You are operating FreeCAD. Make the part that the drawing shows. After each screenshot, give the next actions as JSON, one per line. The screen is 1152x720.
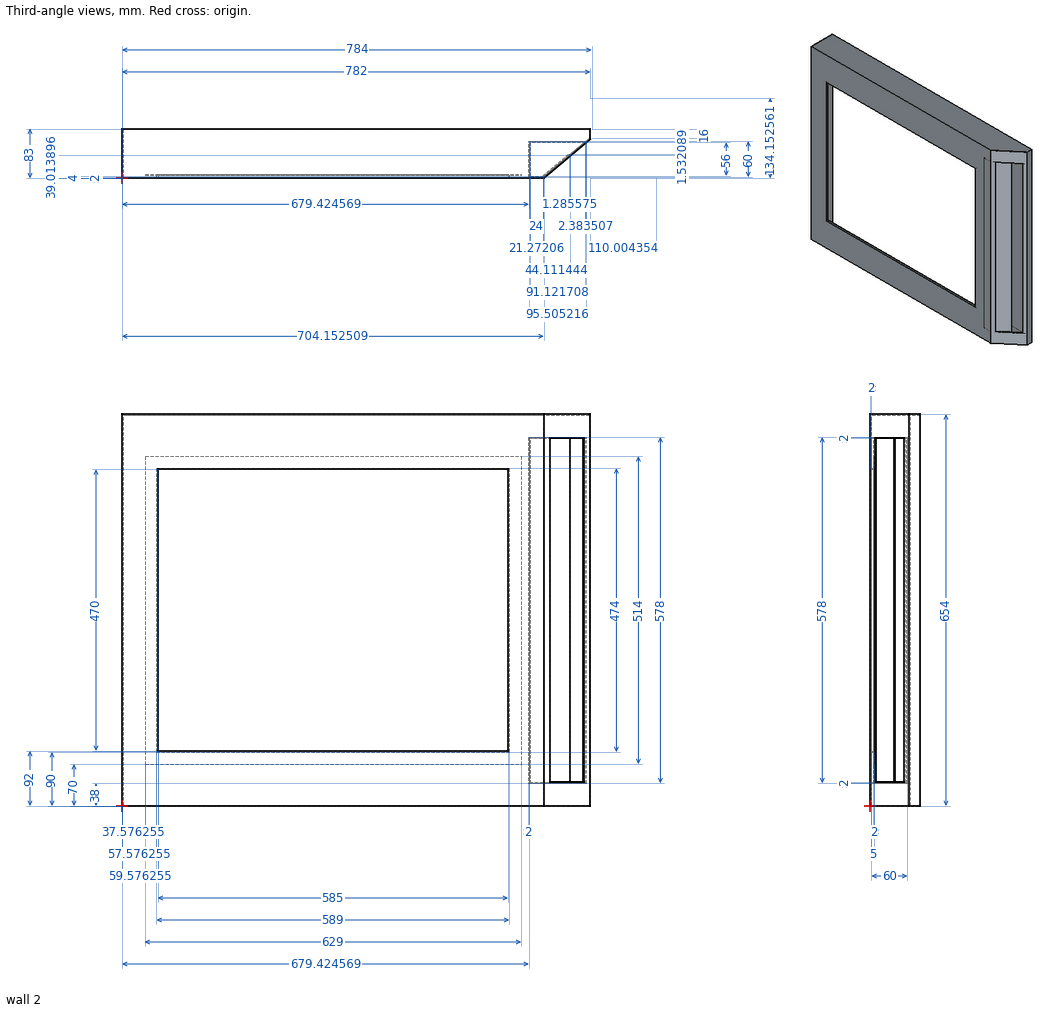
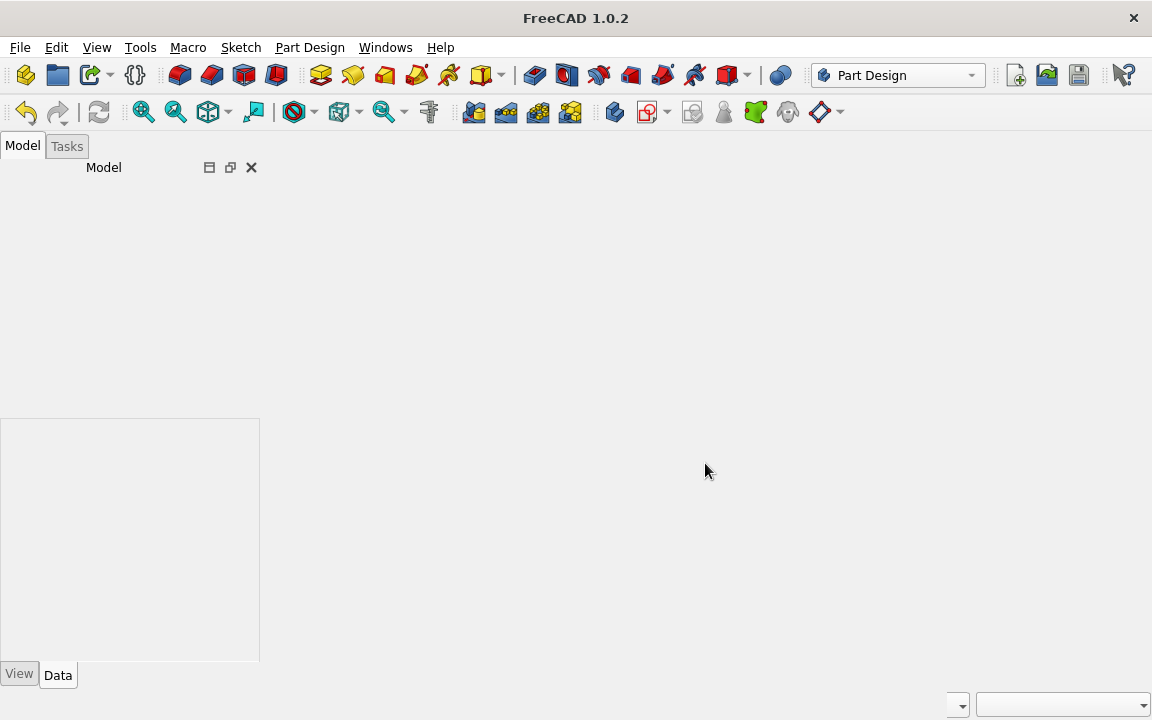
{"action": "key", "text": "ctrl+n"}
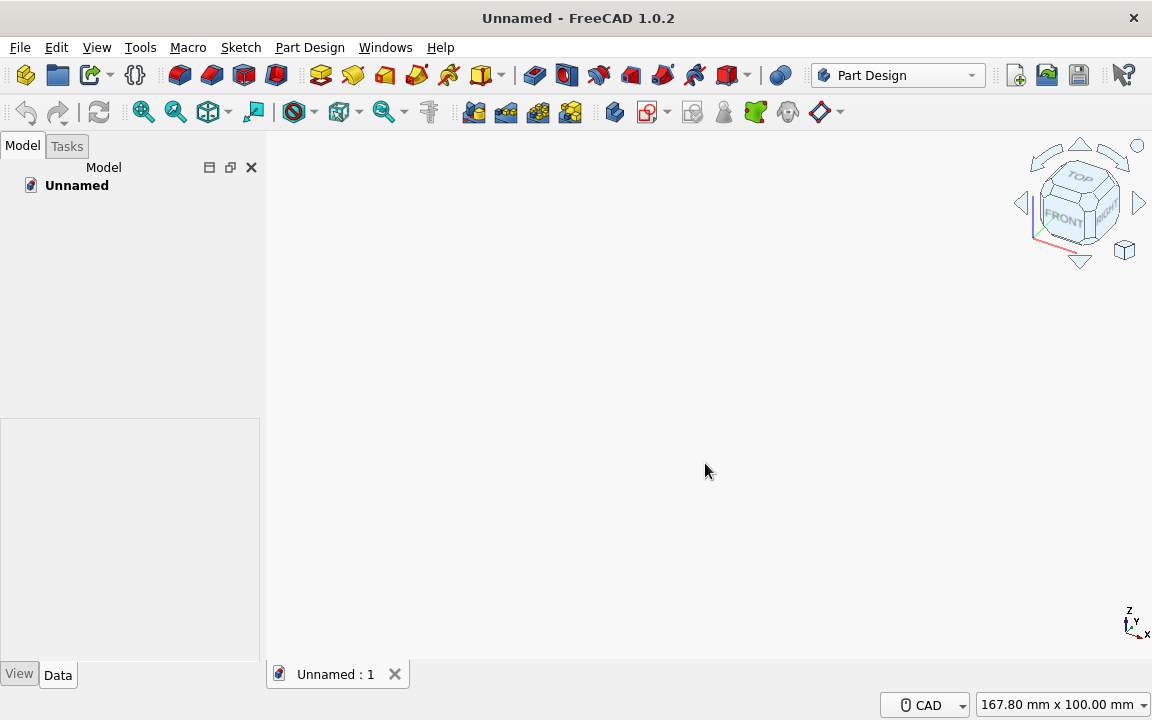
{"action": "left_click", "coordinate": [648, 112]}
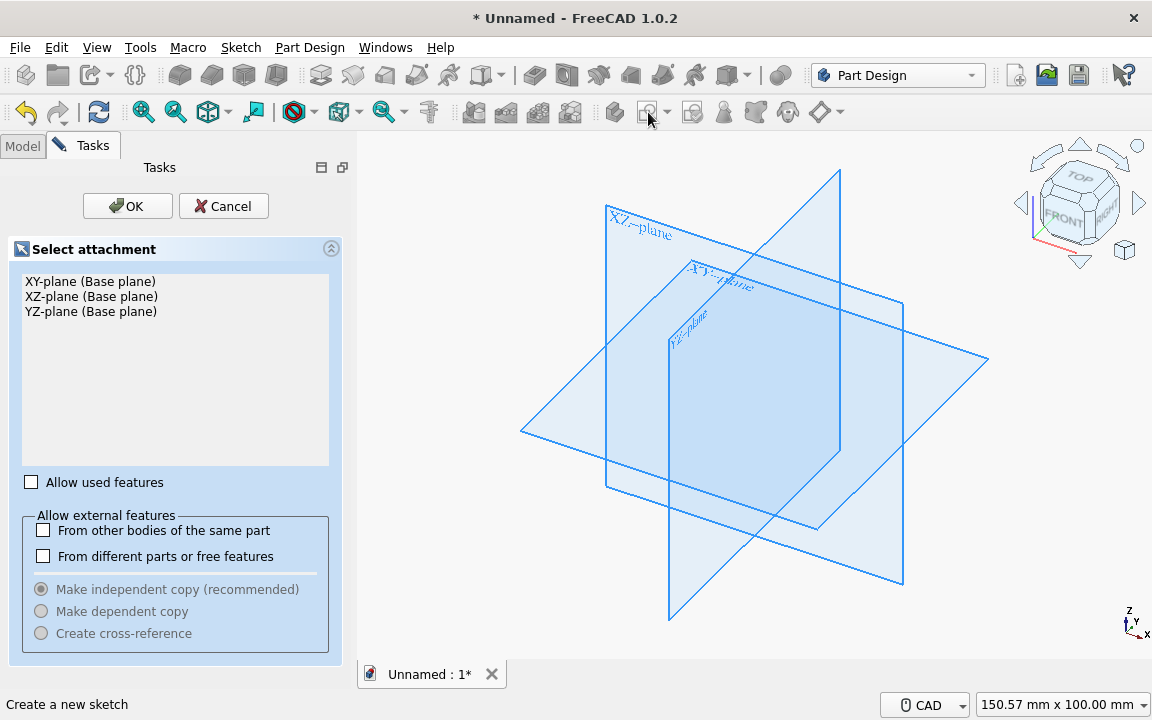
{"action": "left_click", "coordinate": [82, 282]}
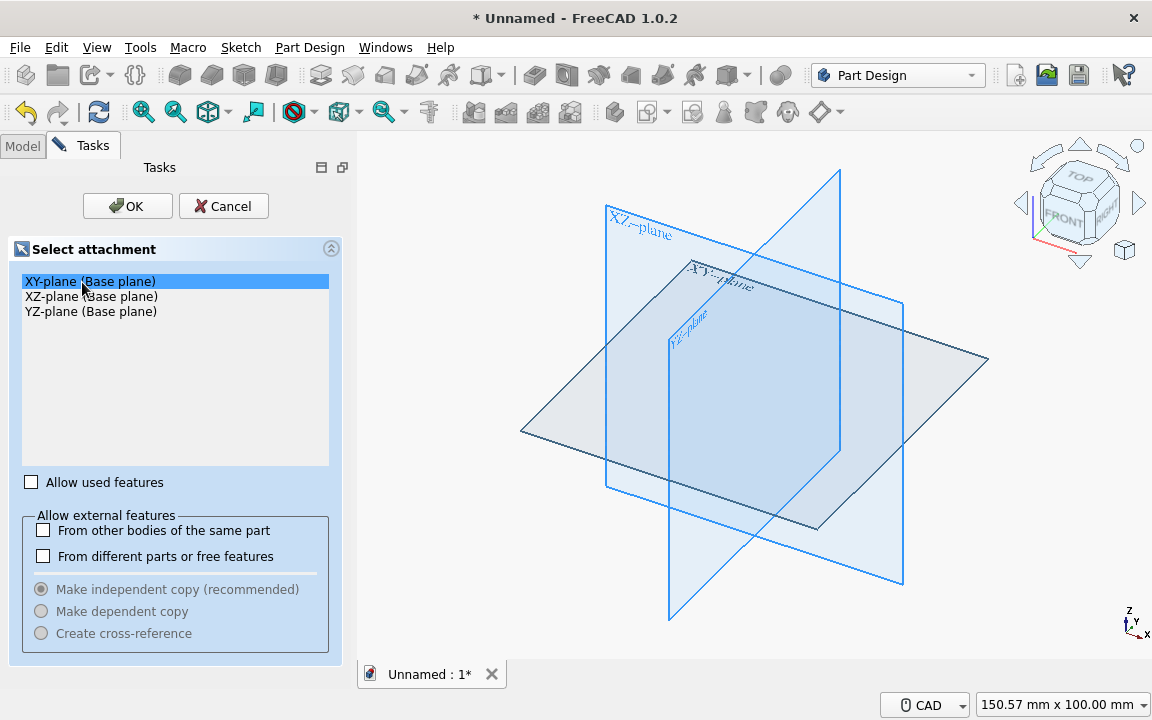
{"action": "left_click", "coordinate": [128, 206]}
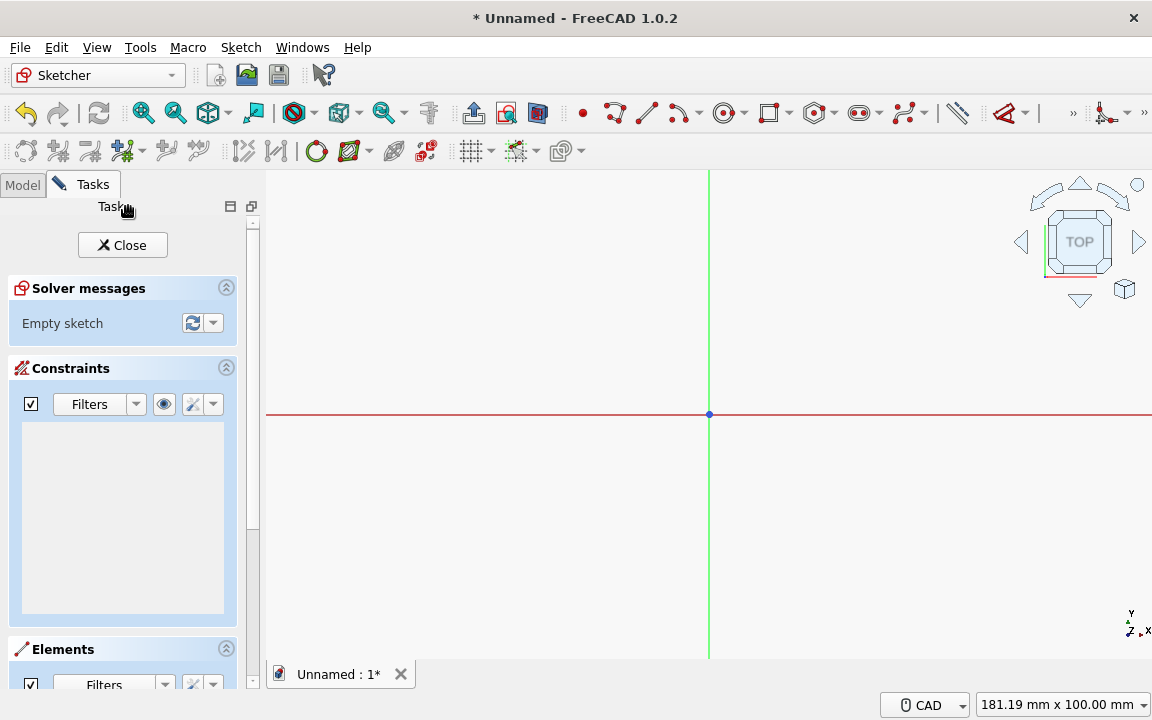
{"action": "scroll", "coordinate": [330, 446], "scroll_direction": "down", "scroll_amount": 10}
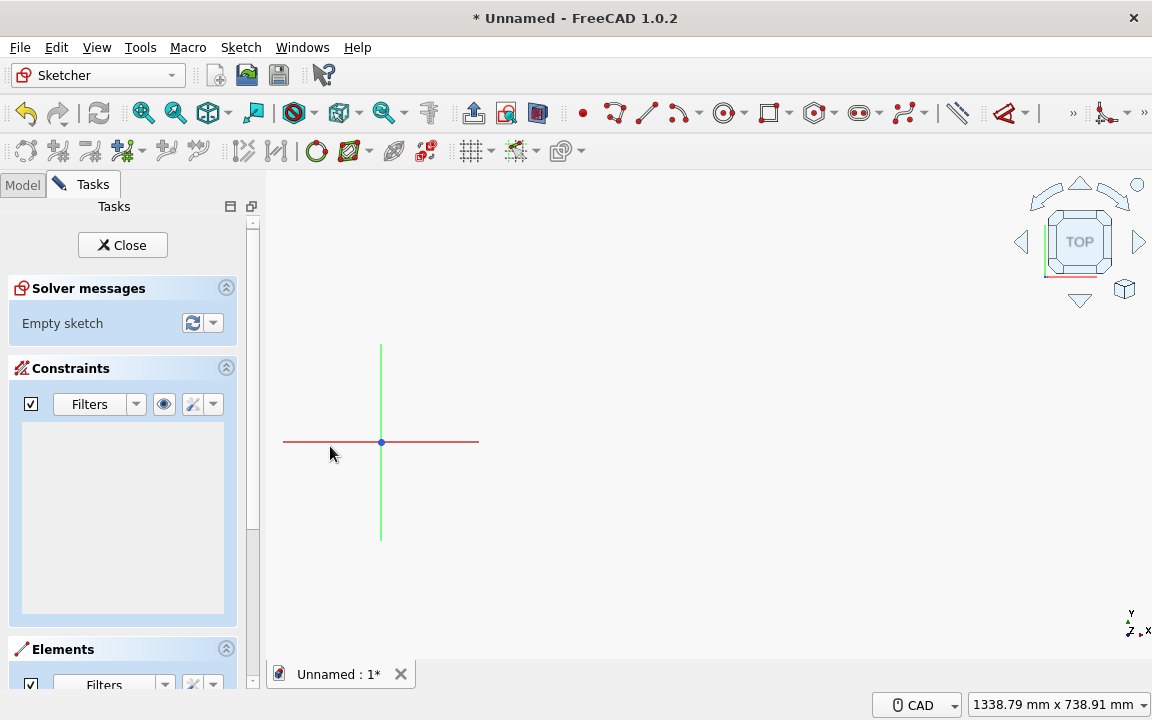
{"action": "key", "text": "g m"}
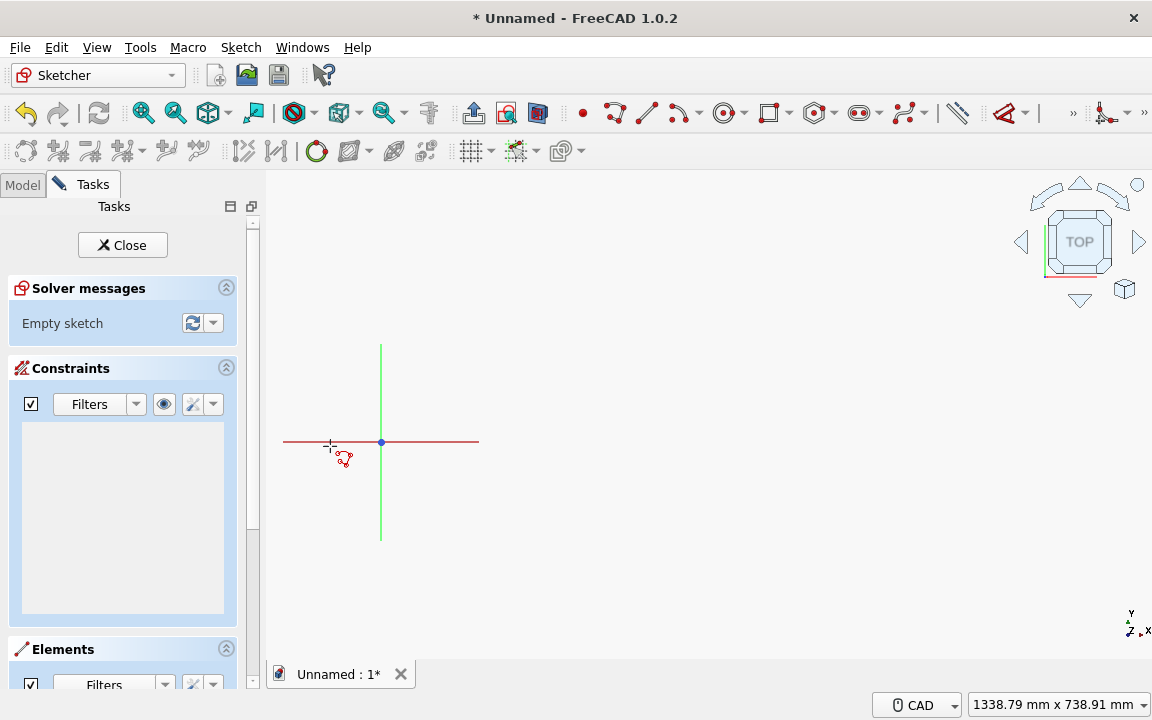
{"action": "left_click", "coordinate": [381, 442]}
{"action": "left_click", "coordinate": [847, 433]}
{"action": "left_click", "coordinate": [900, 398]}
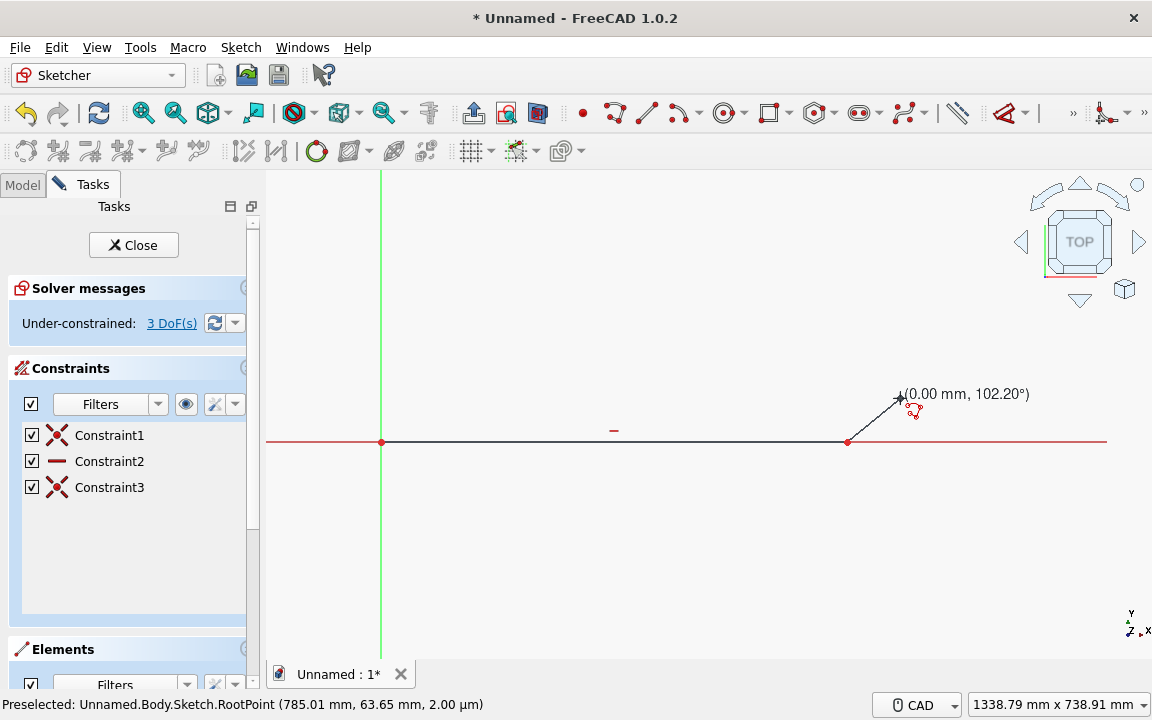
{"action": "scroll", "coordinate": [900, 387], "scroll_direction": "up", "scroll_amount": 3}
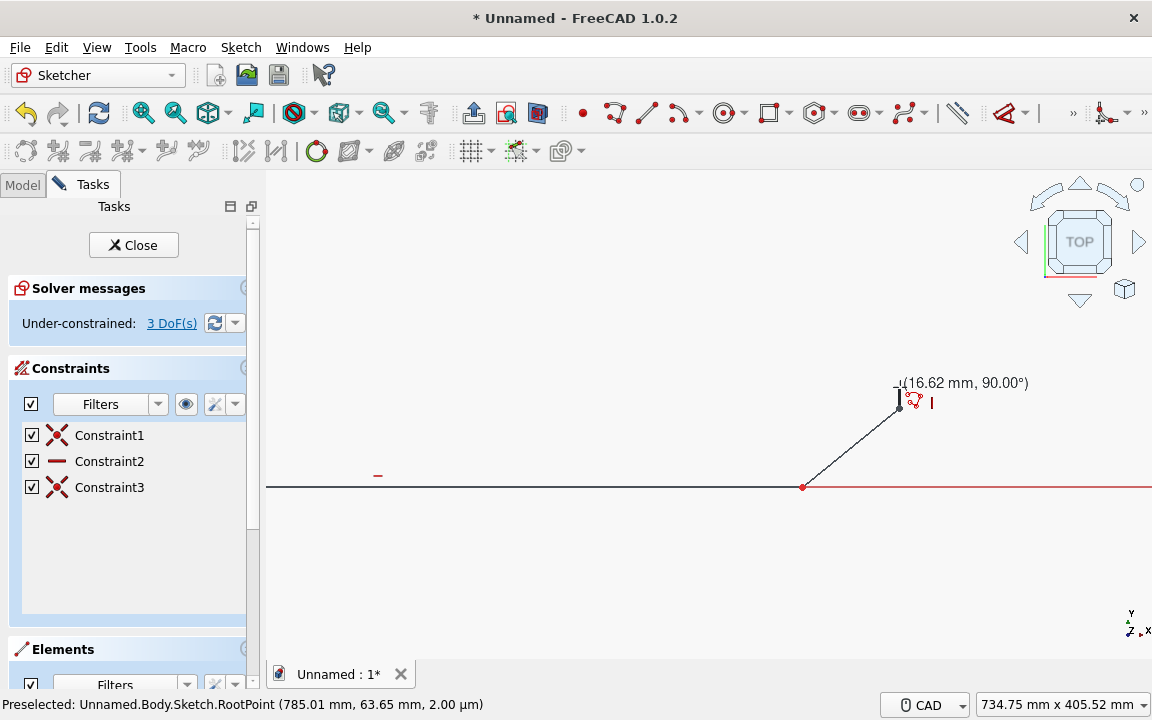
{"action": "left_click", "coordinate": [899, 387]}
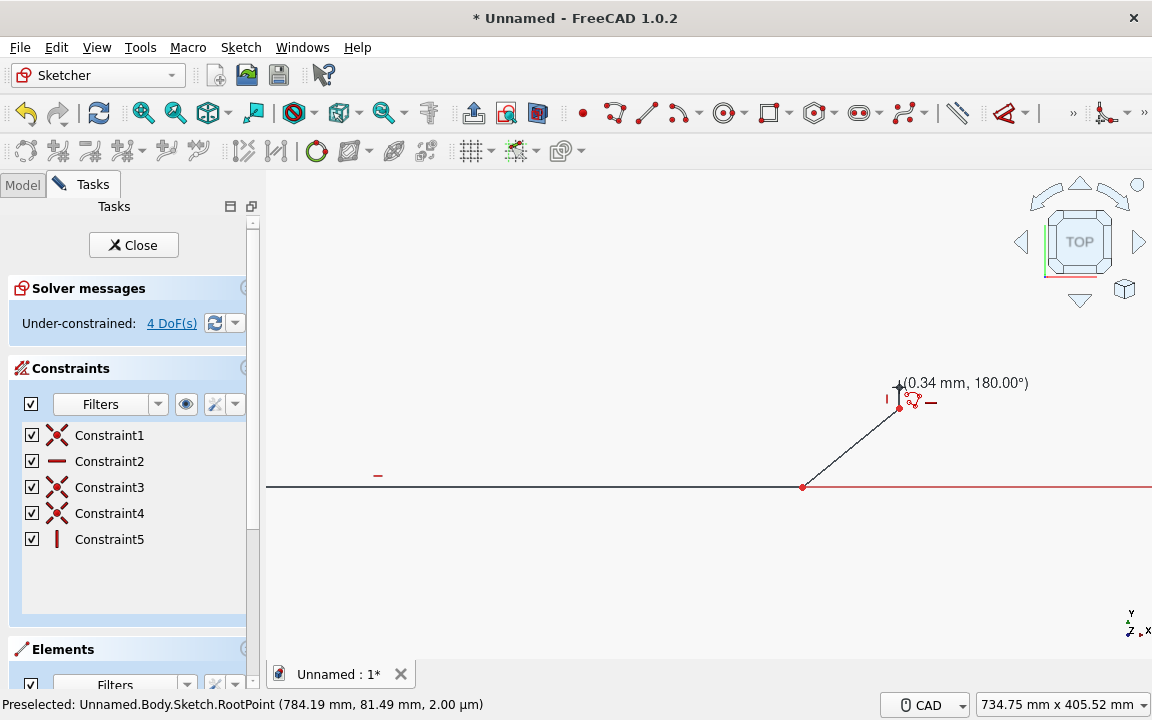
{"action": "scroll", "coordinate": [900, 387], "scroll_direction": "down", "scroll_amount": 3}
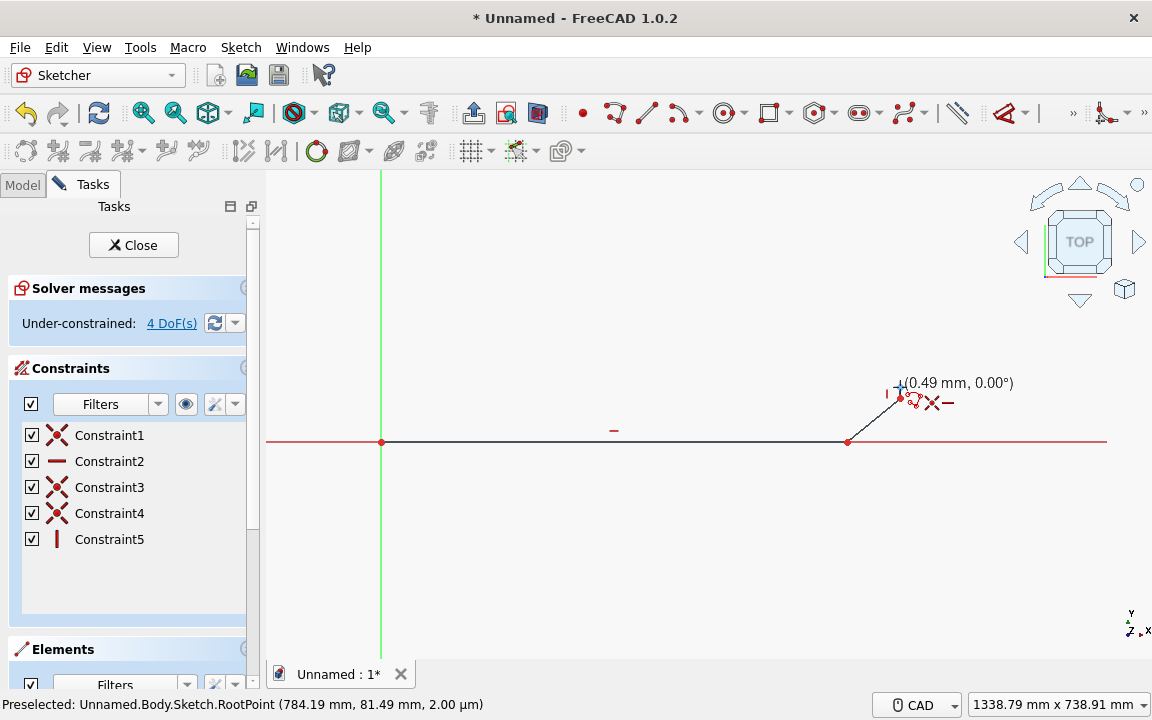
{"action": "left_click", "coordinate": [390, 387]}
{"action": "left_click", "coordinate": [381, 442]}
{"action": "key", "text": "Escape"}
{"action": "key", "text": "Escape"}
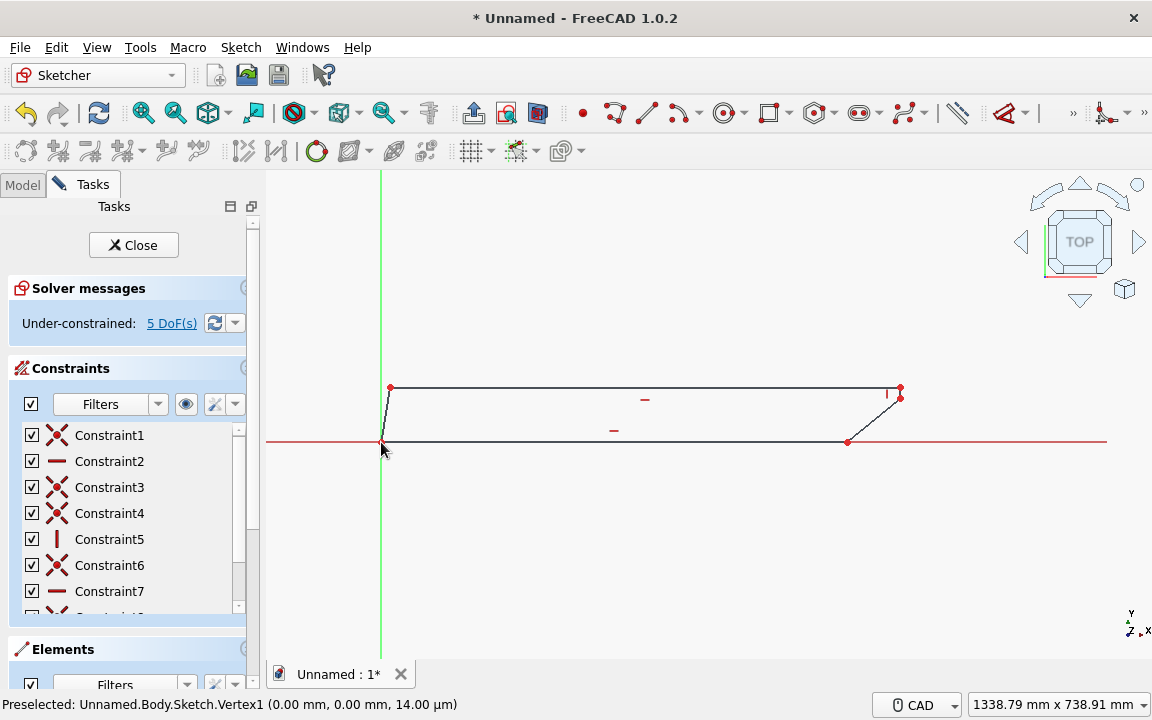
{"action": "left_click", "coordinate": [384, 426]}